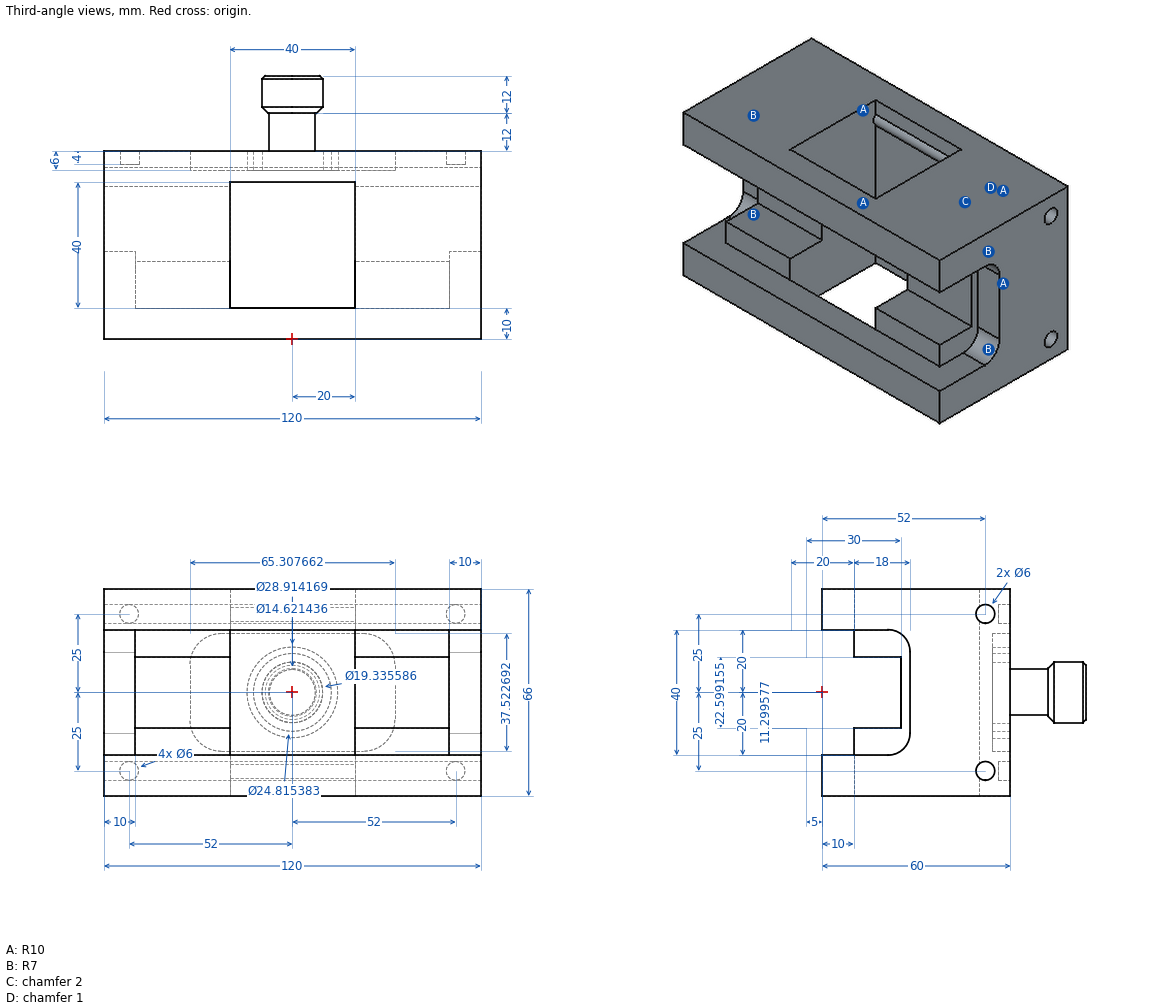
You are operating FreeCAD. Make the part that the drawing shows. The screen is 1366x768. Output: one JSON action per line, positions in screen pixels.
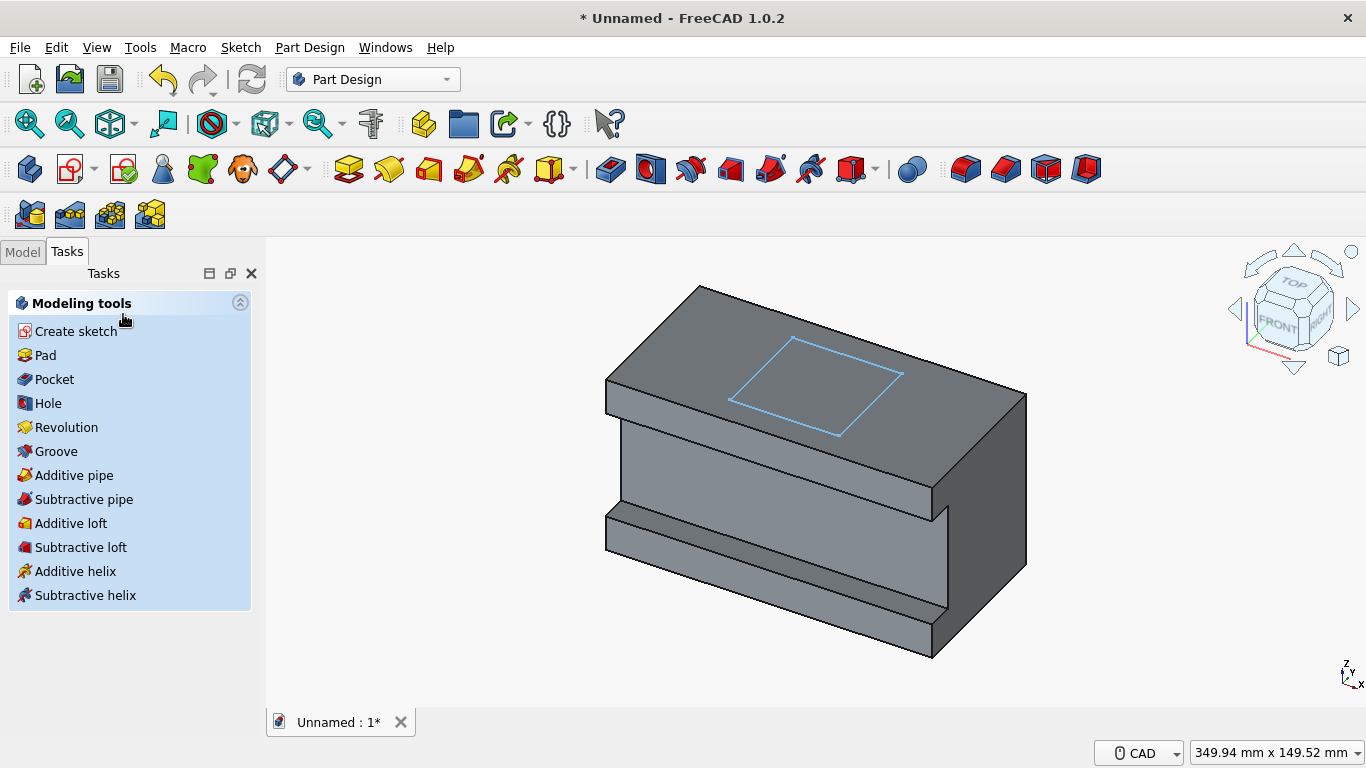
{"action": "left_click", "coordinate": [612, 170]}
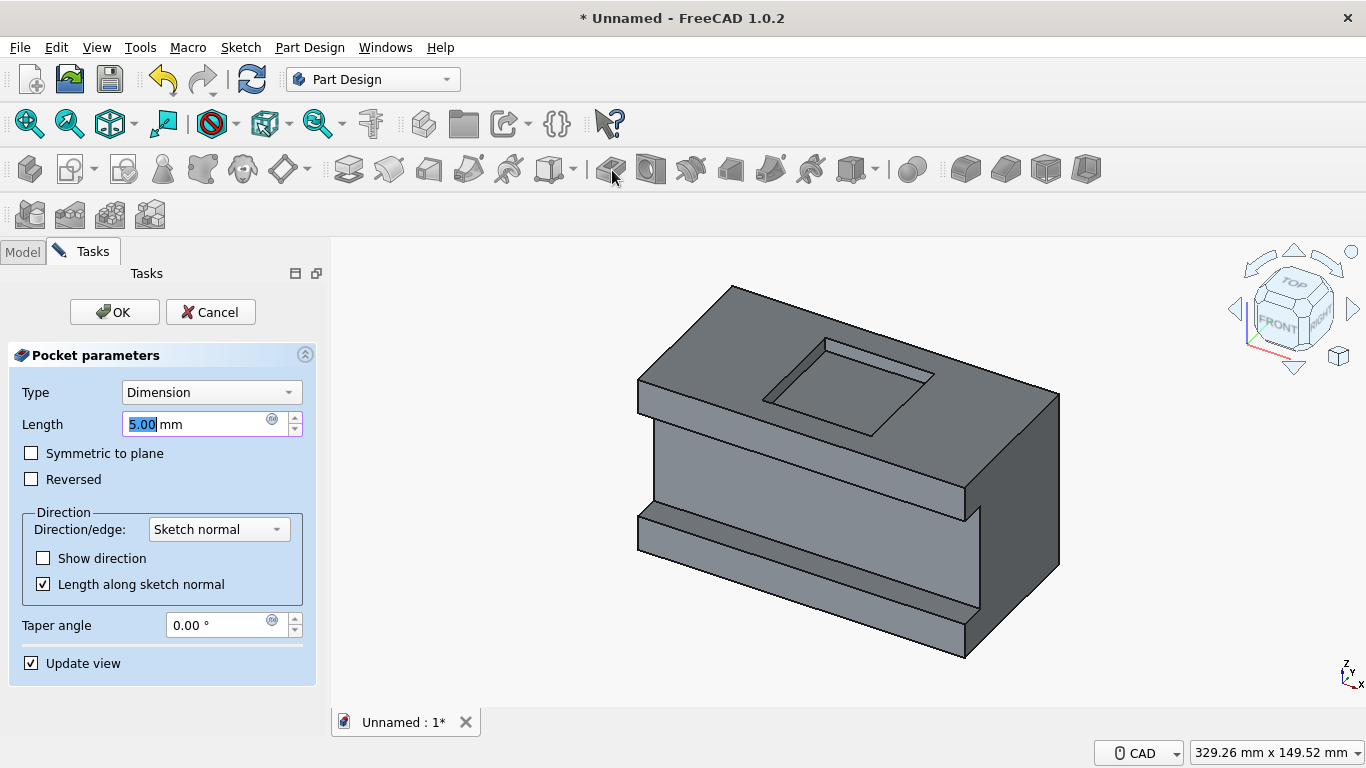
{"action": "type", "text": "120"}
{"action": "key", "text": "Tab"}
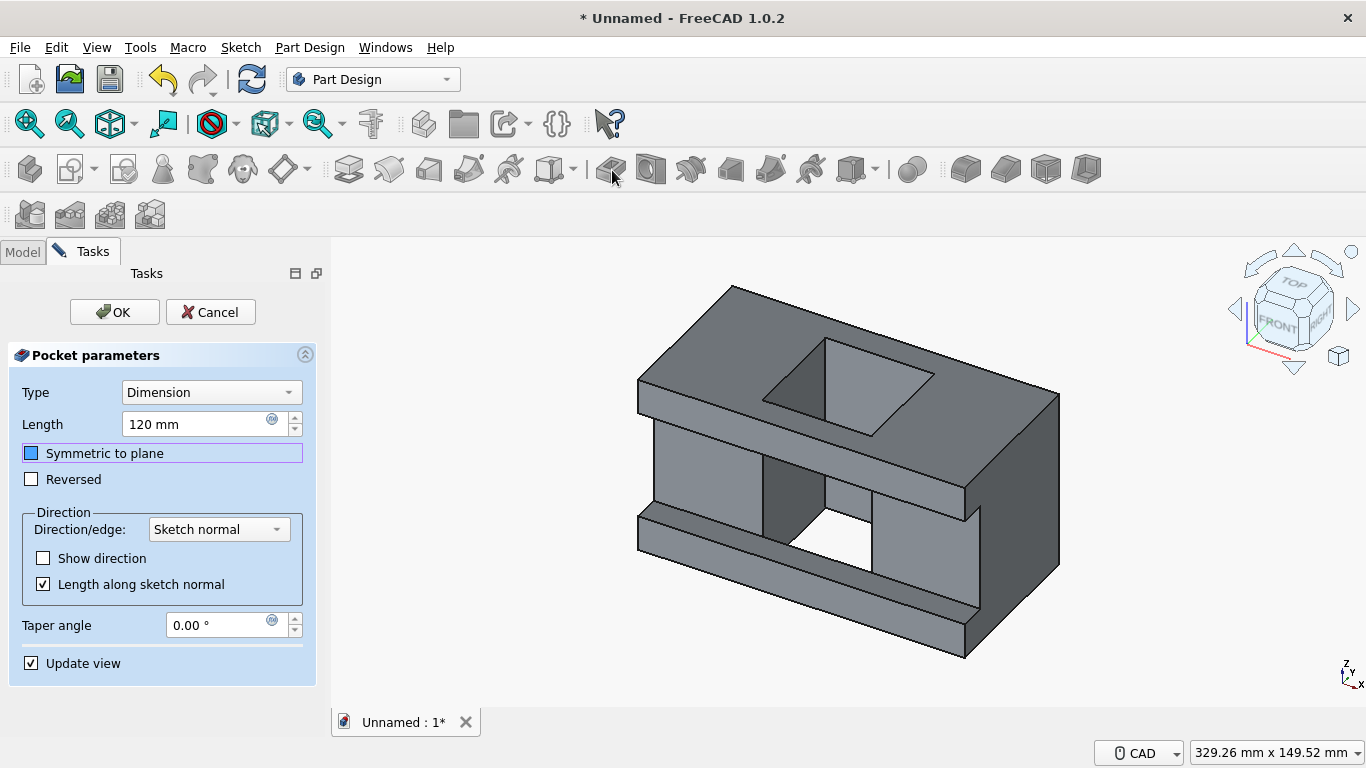
{"action": "left_click", "coordinate": [115, 312]}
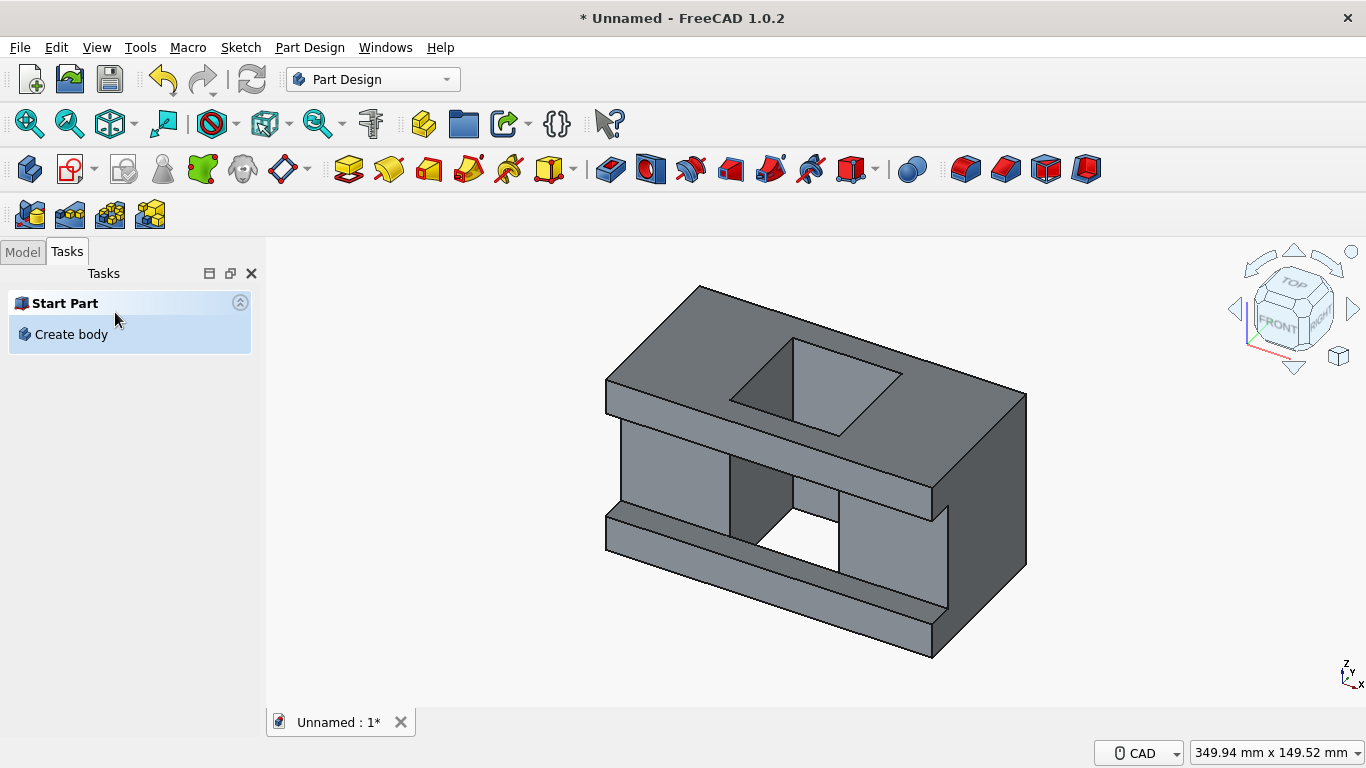
{"action": "left_click", "coordinate": [993, 536]}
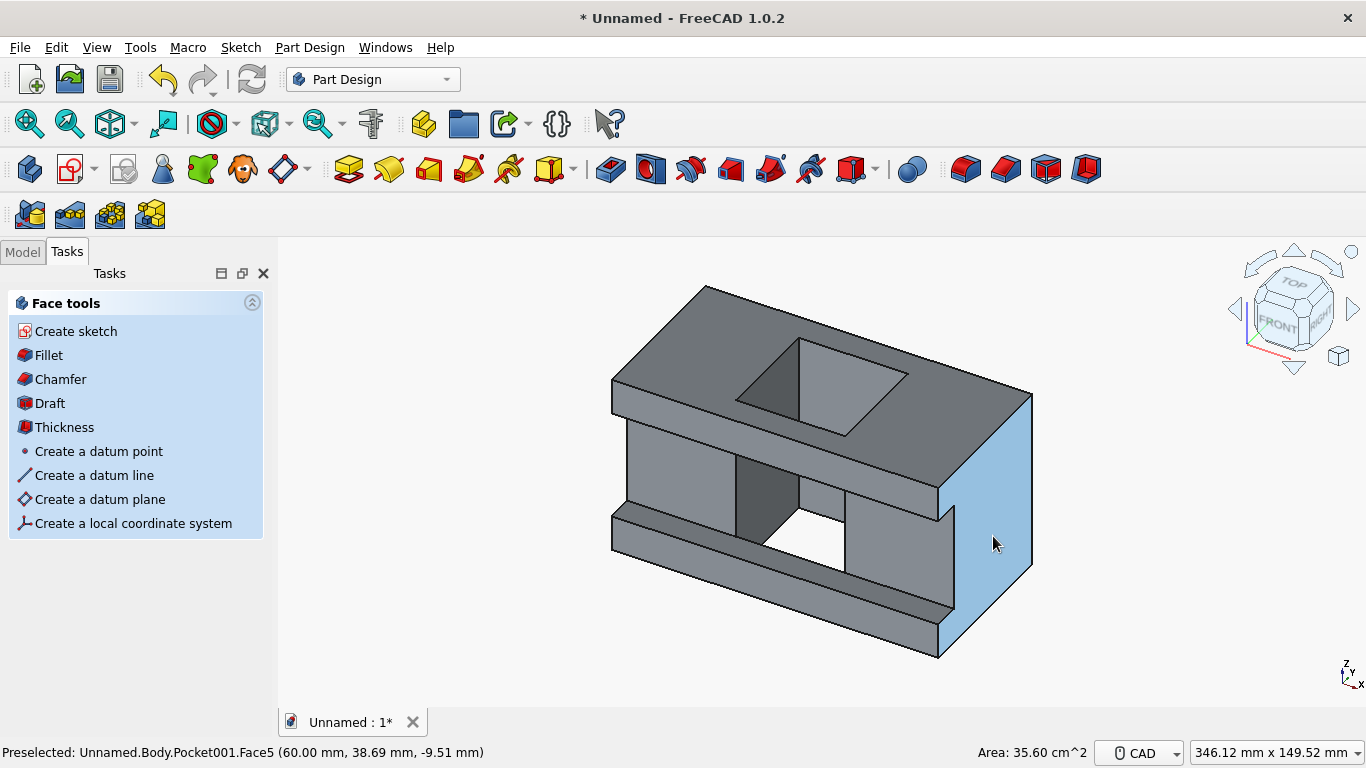
{"action": "left_click", "coordinate": [70, 170]}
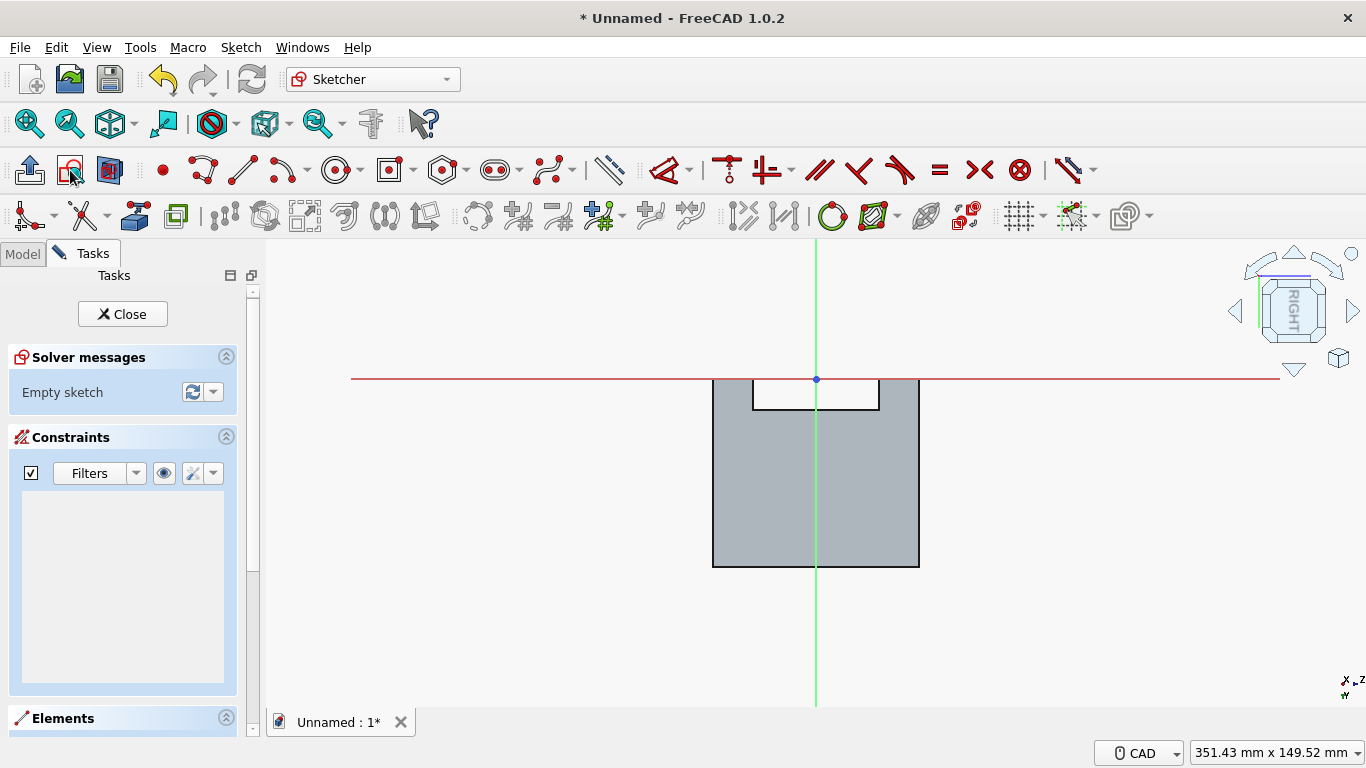
{"action": "scroll", "coordinate": [846, 383], "scroll_direction": "up", "scroll_amount": 6}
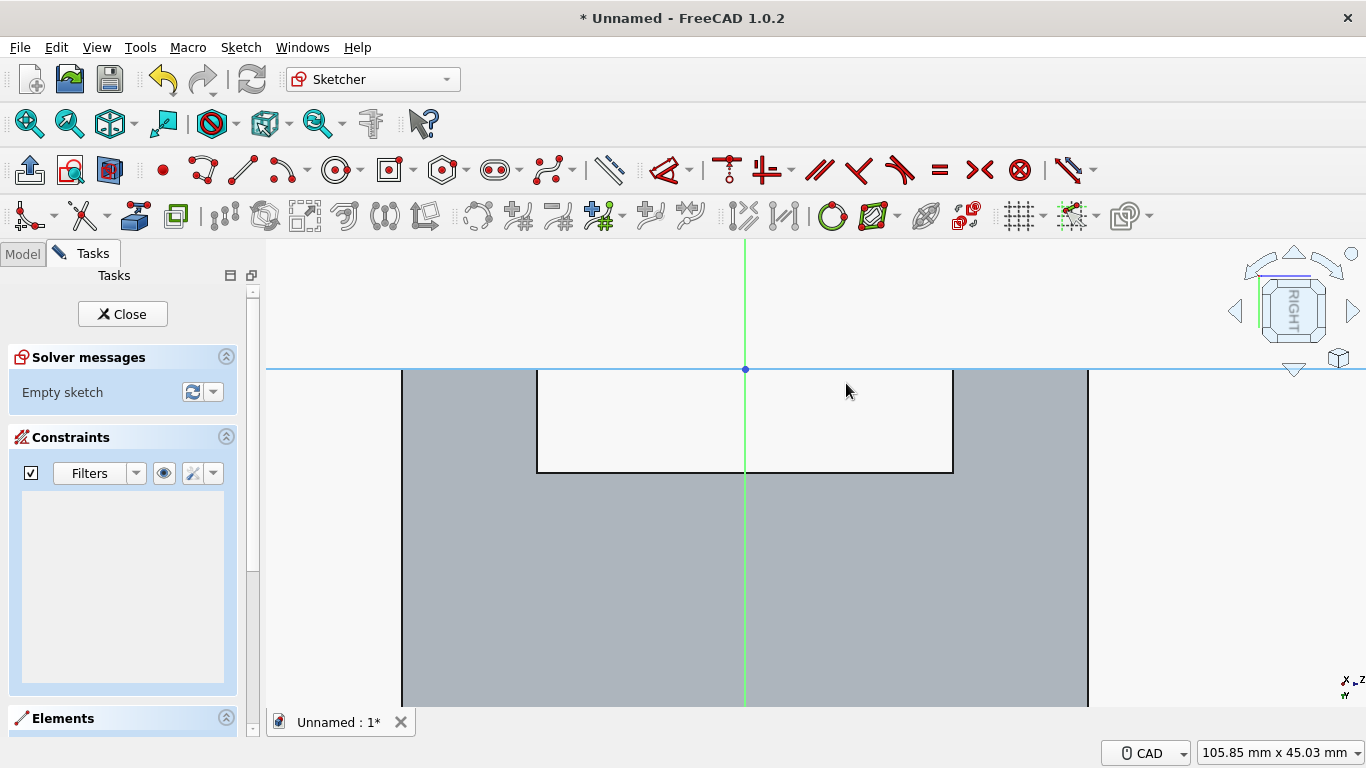
{"action": "key", "text": "g r"}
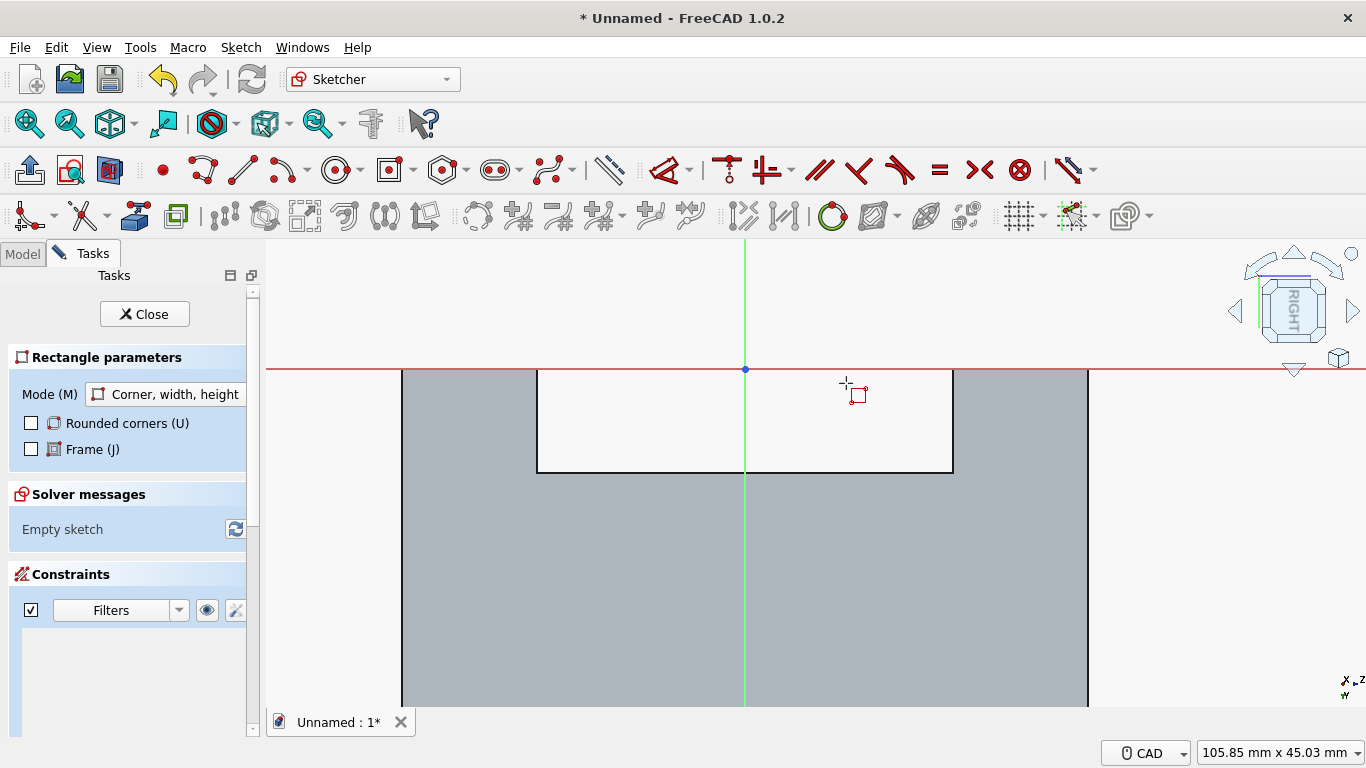
{"action": "left_click", "coordinate": [628, 317]}
{"action": "mouse_move", "coordinate": [863, 629]}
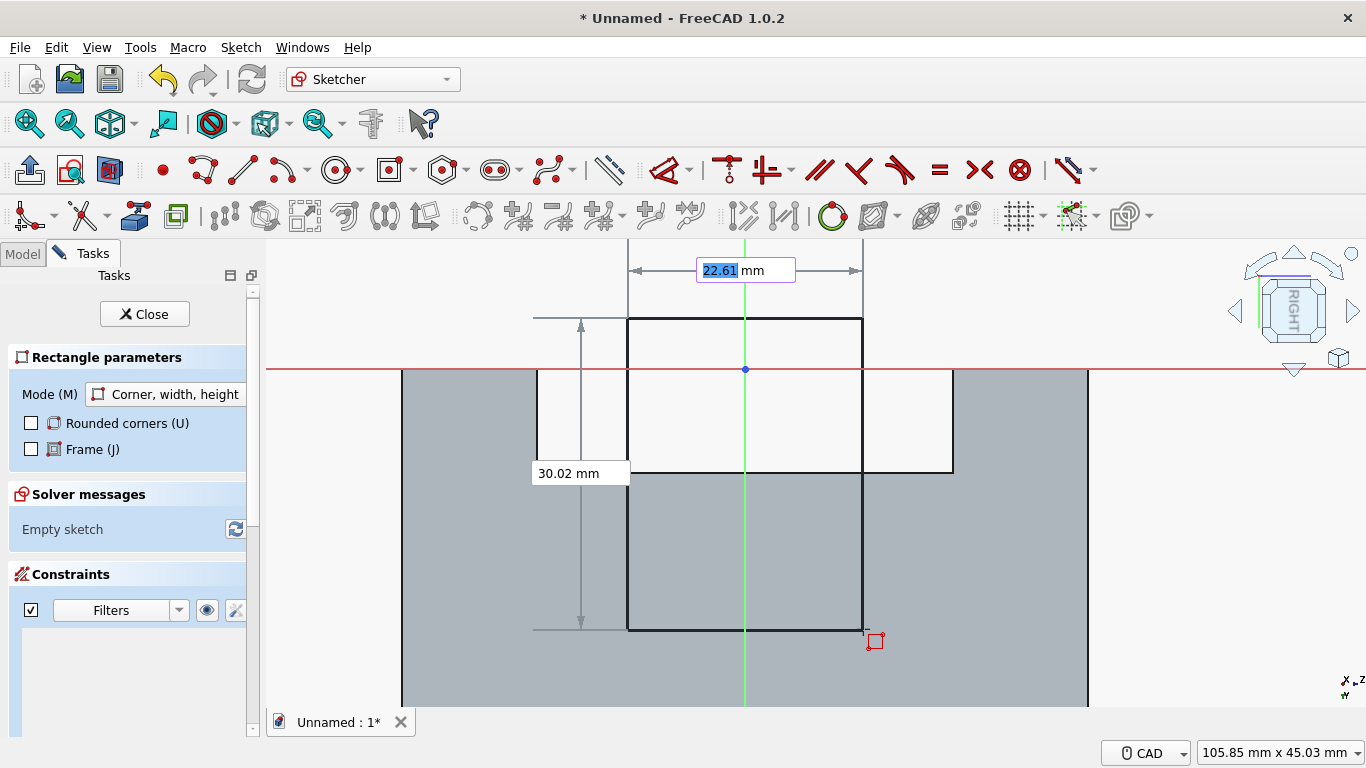
{"action": "type", "text": "22.599155"}
{"action": "key", "text": "Tab"}
{"action": "type", "text": "30"}
{"action": "key", "text": "Return"}
{"action": "key", "text": "Escape"}